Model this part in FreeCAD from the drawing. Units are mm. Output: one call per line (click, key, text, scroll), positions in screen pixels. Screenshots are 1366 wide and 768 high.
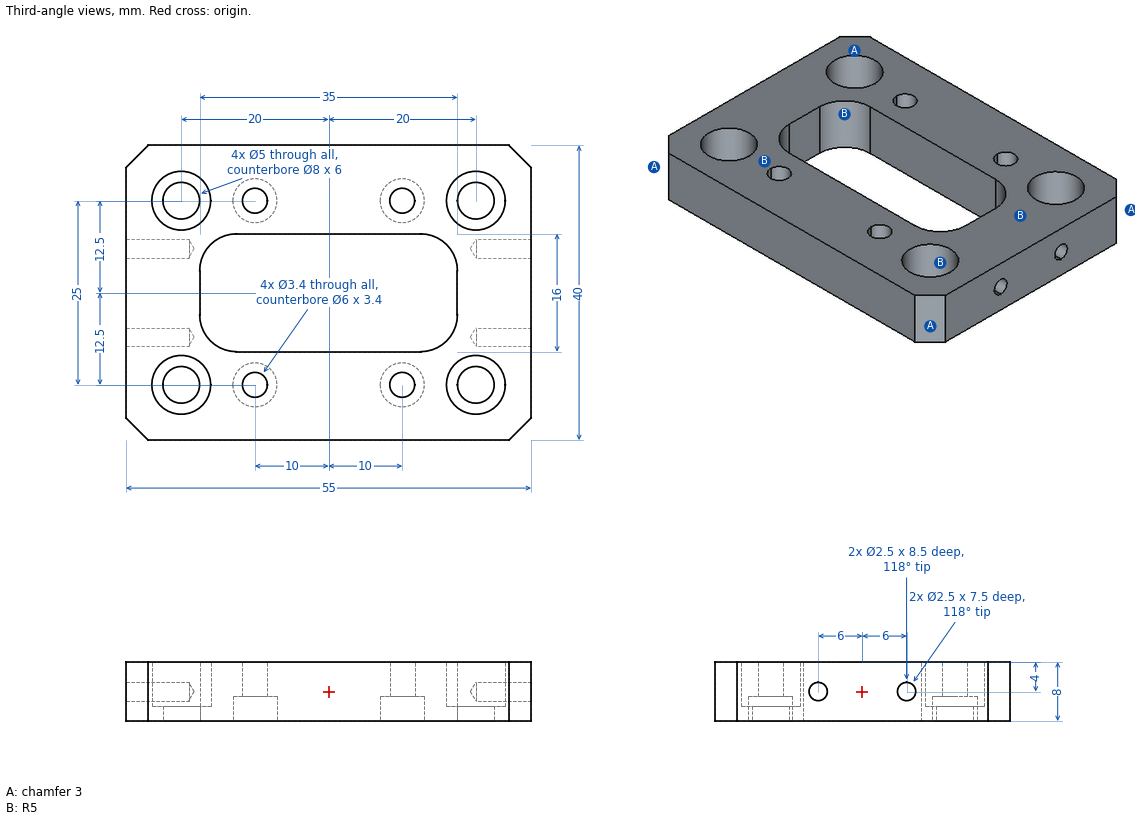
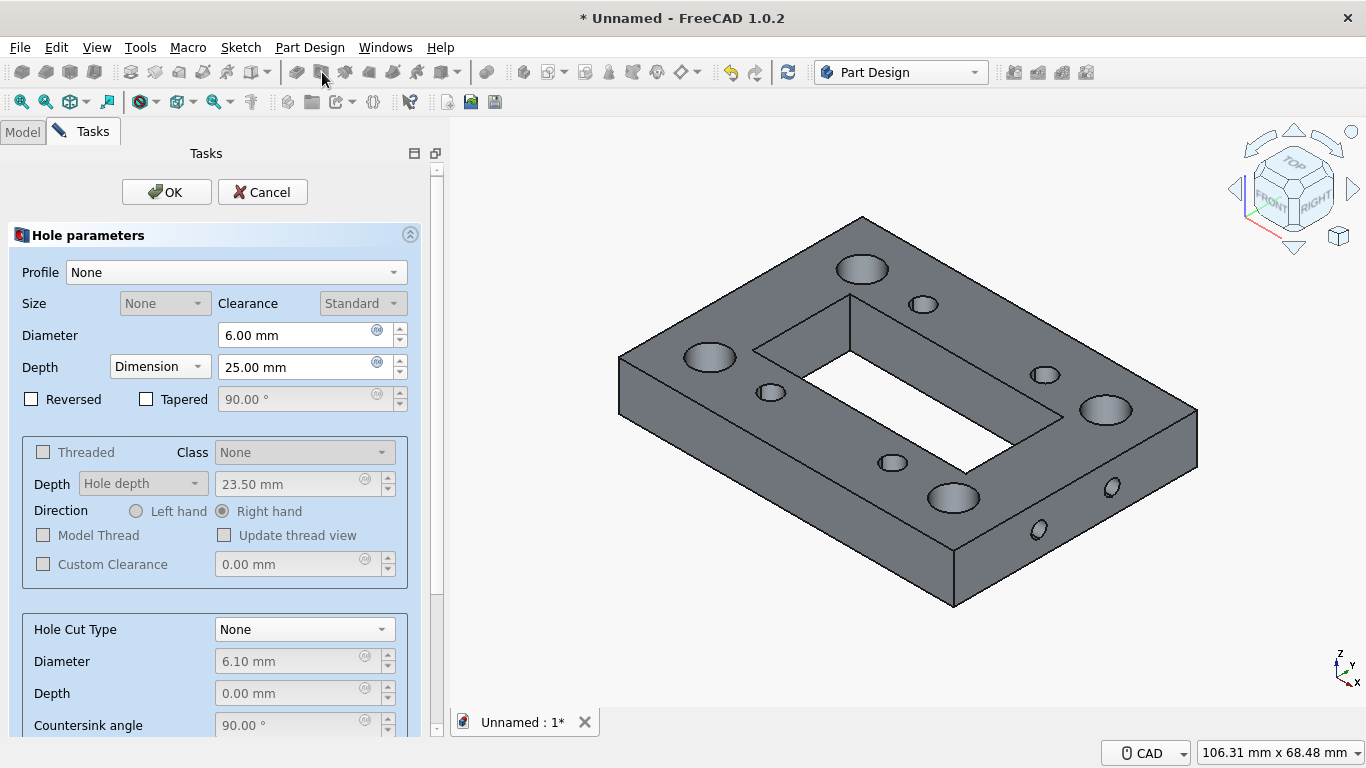
triple_click(305, 335)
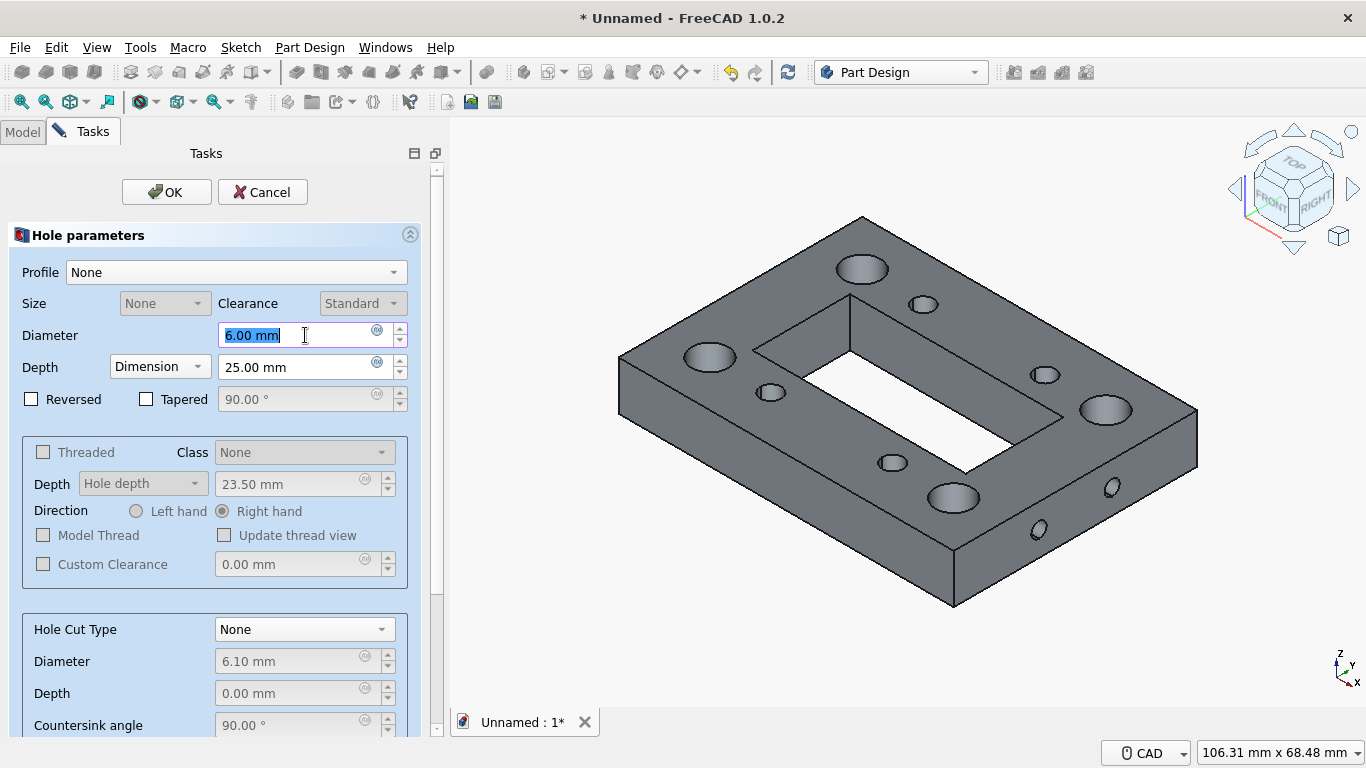
text(5)
key(Tab)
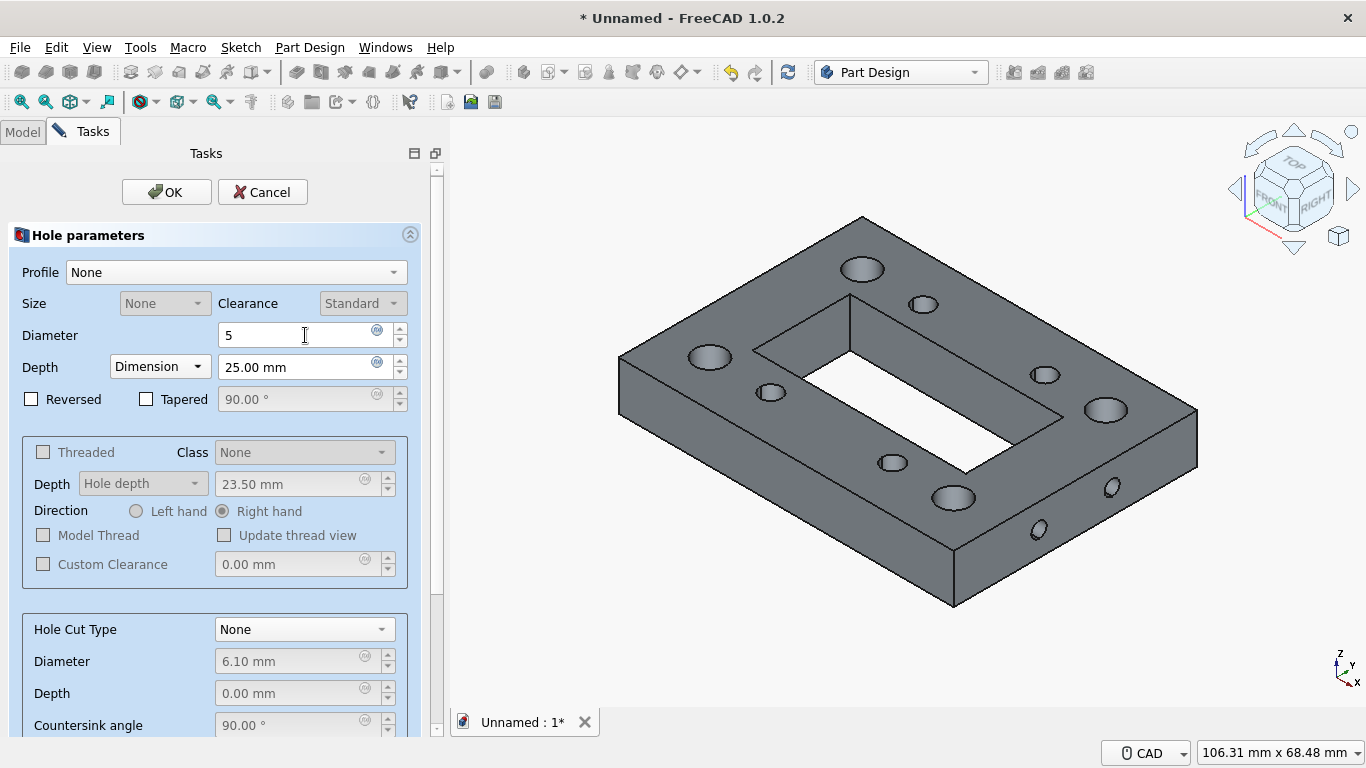
click(161, 366)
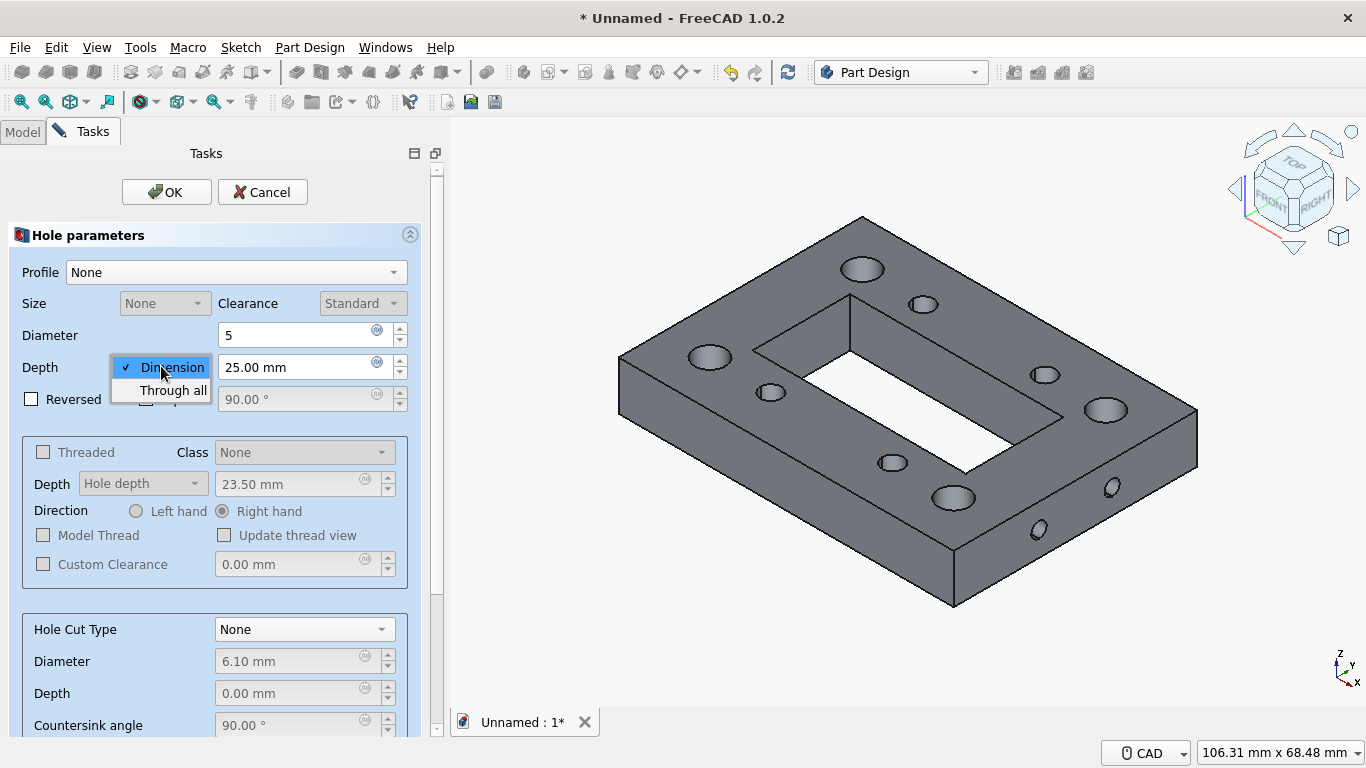
click(160, 390)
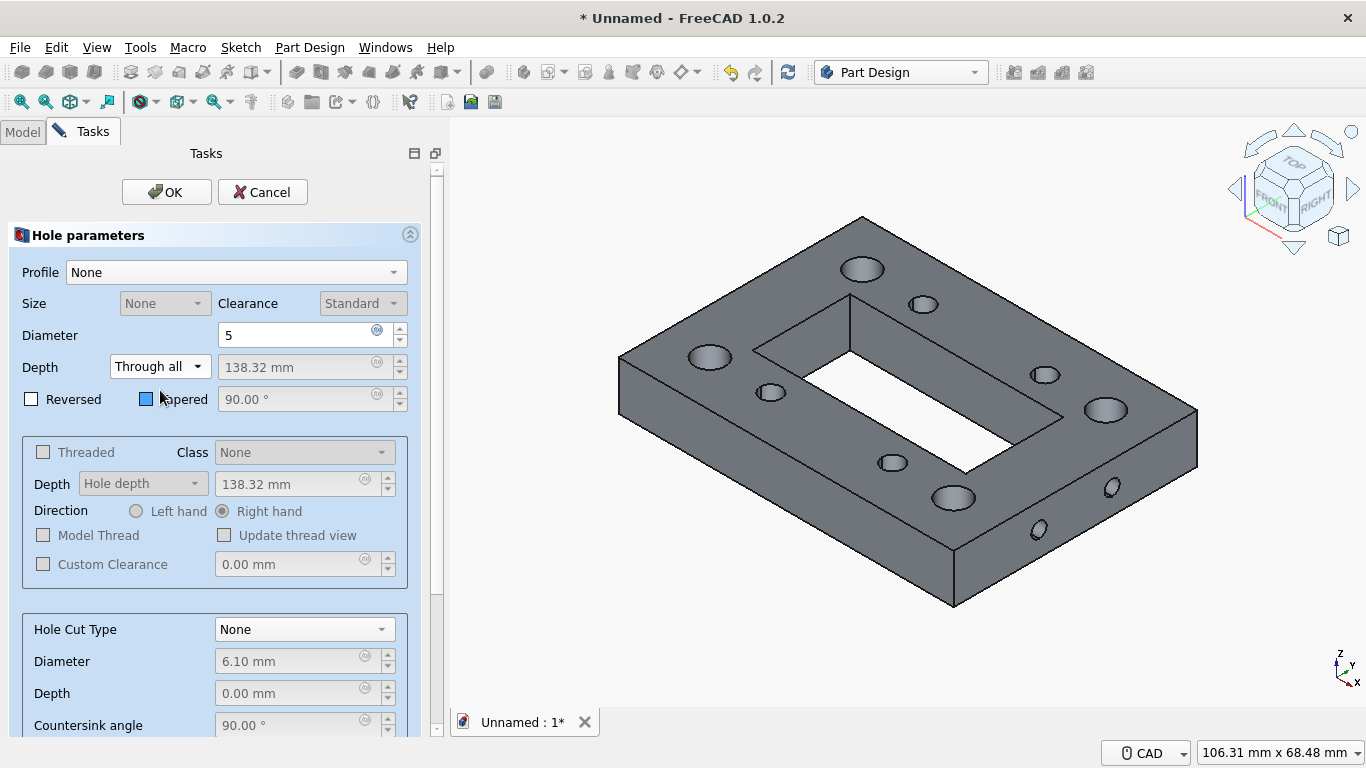
click(306, 630)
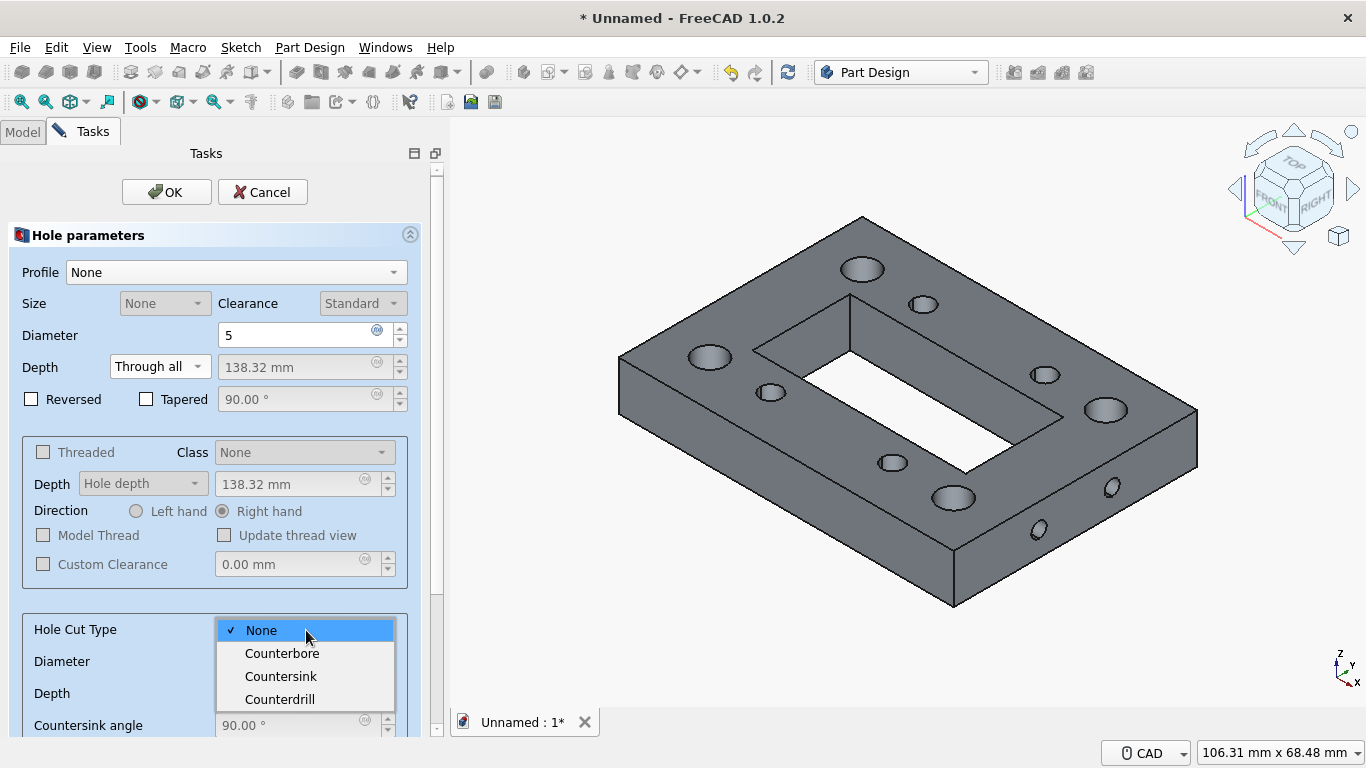
click(304, 654)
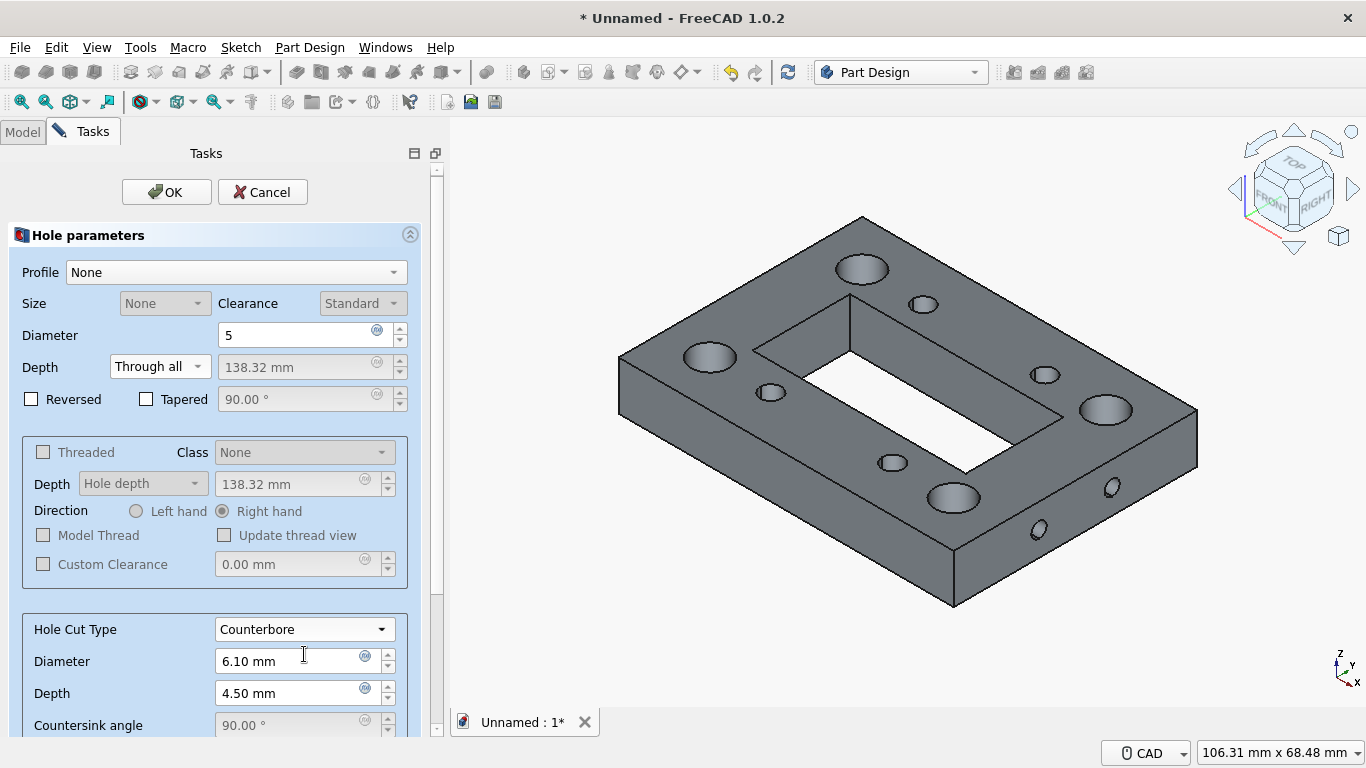
triple_click(298, 661)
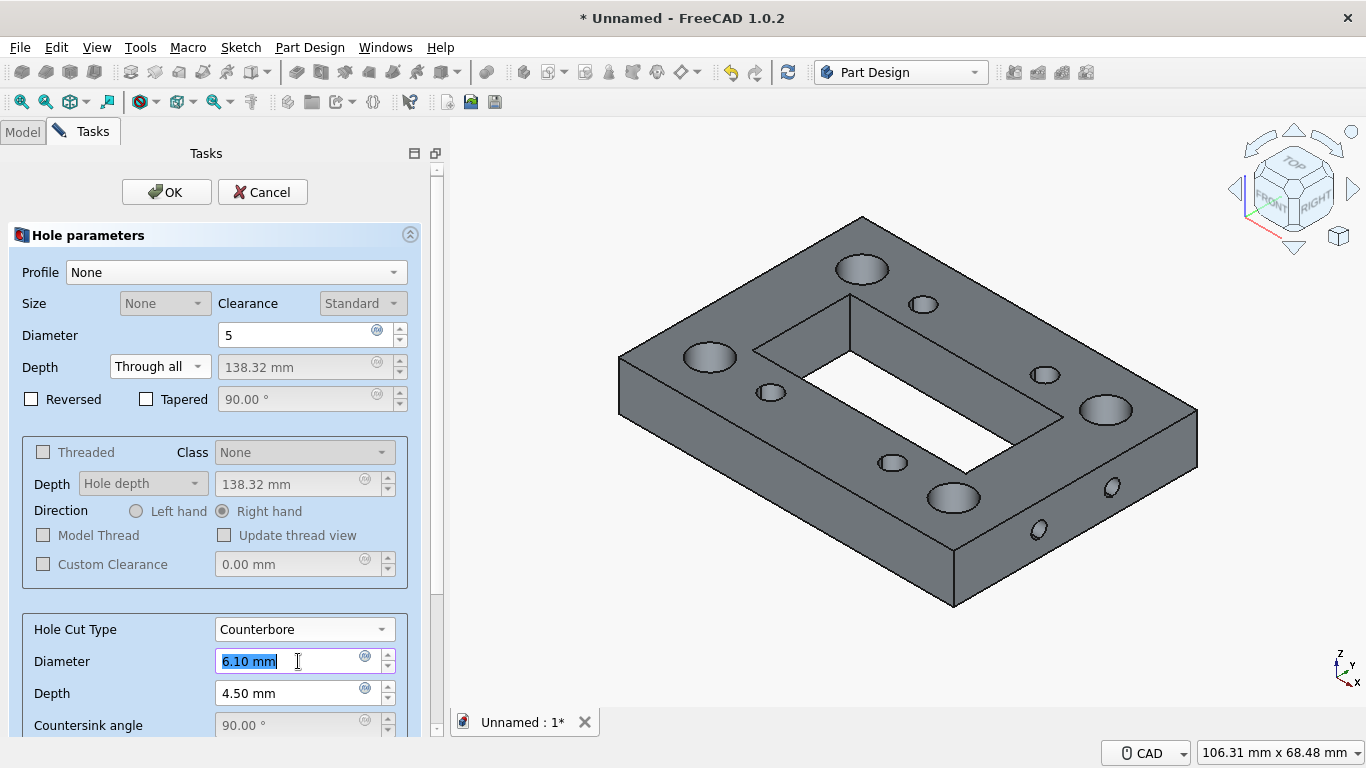
text(8)
key(Tab)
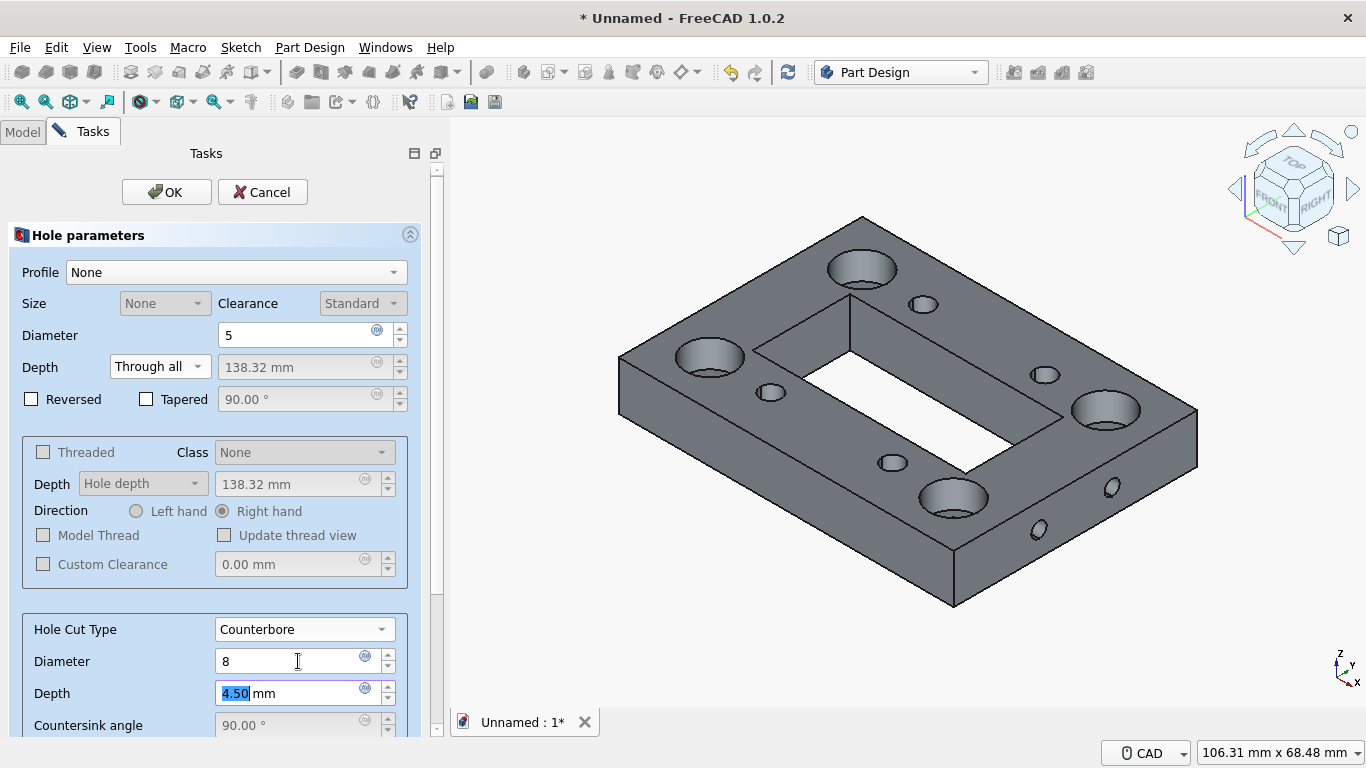
text(6)
key(Tab)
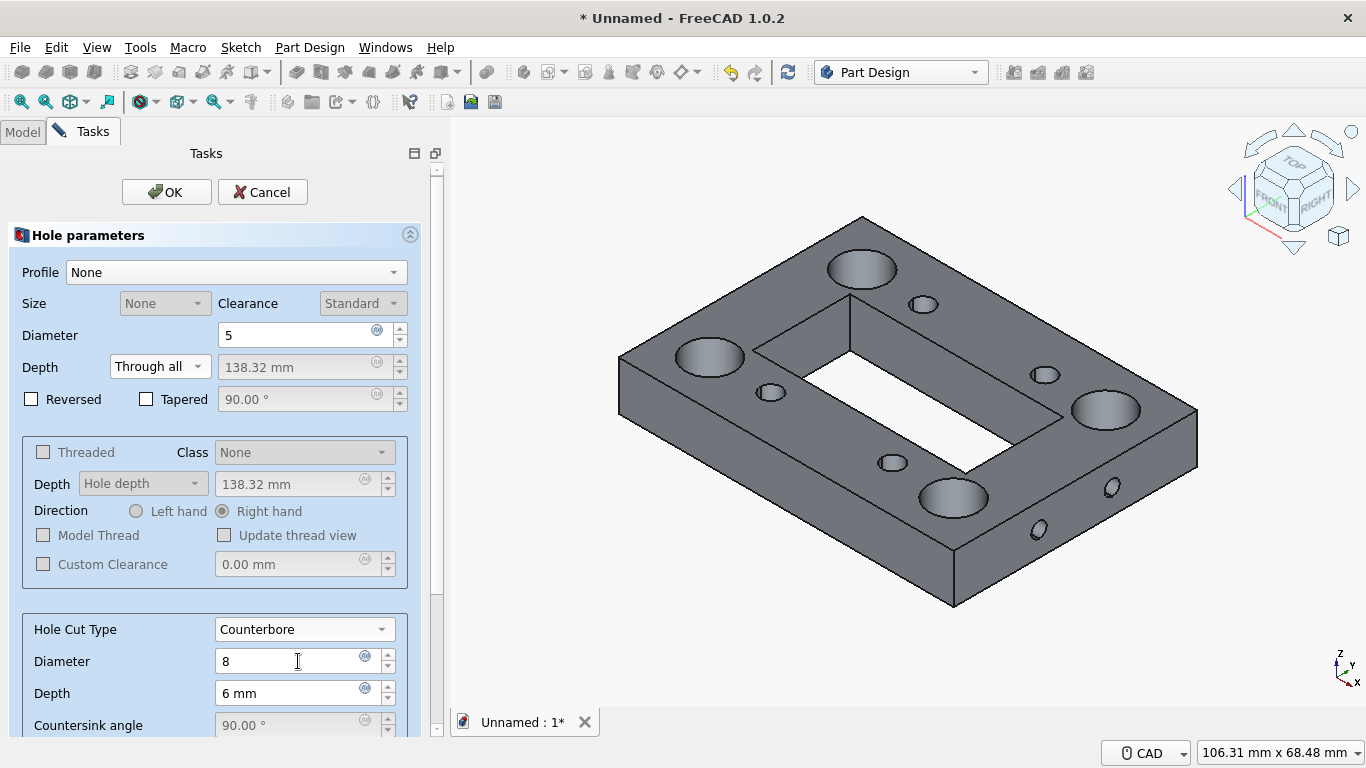
click(167, 192)